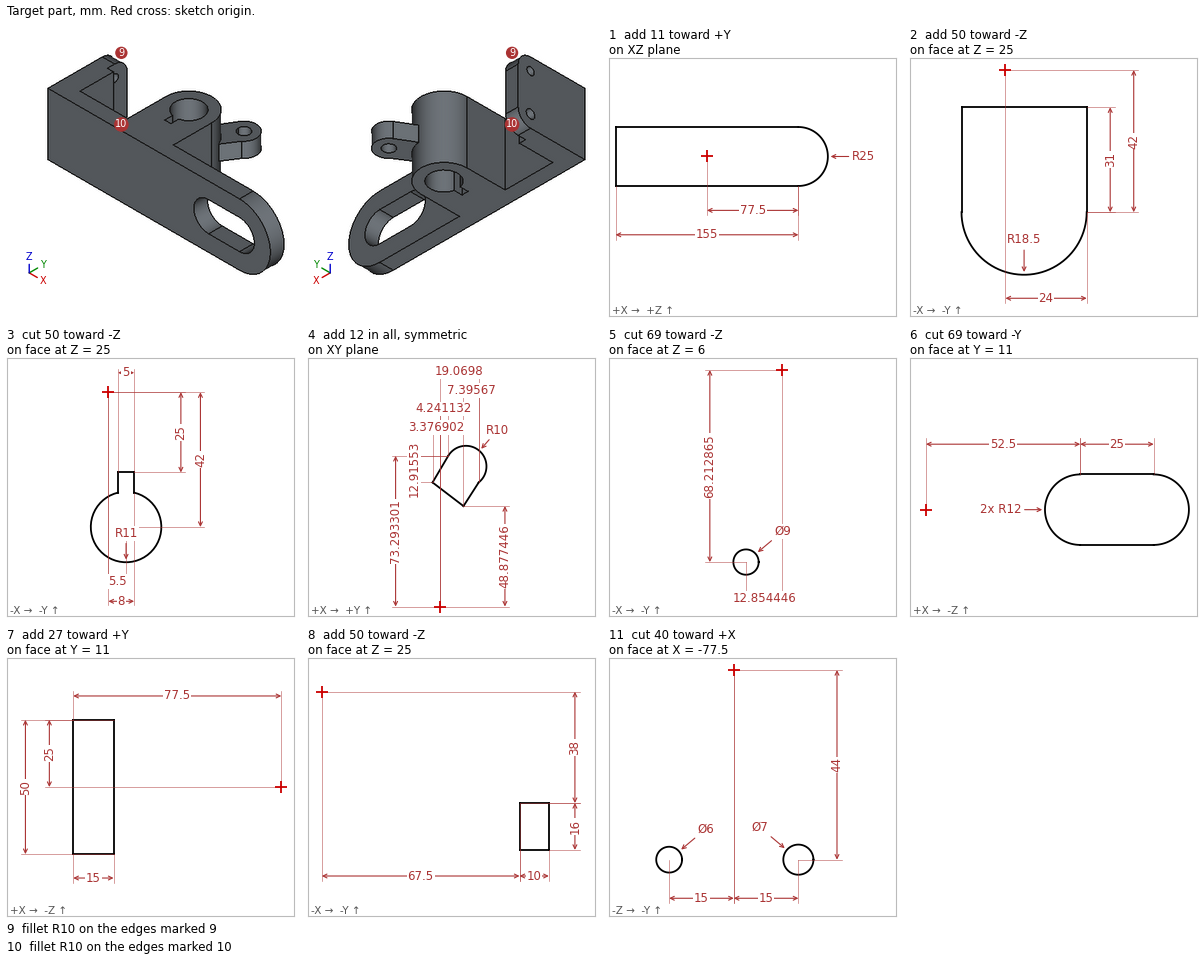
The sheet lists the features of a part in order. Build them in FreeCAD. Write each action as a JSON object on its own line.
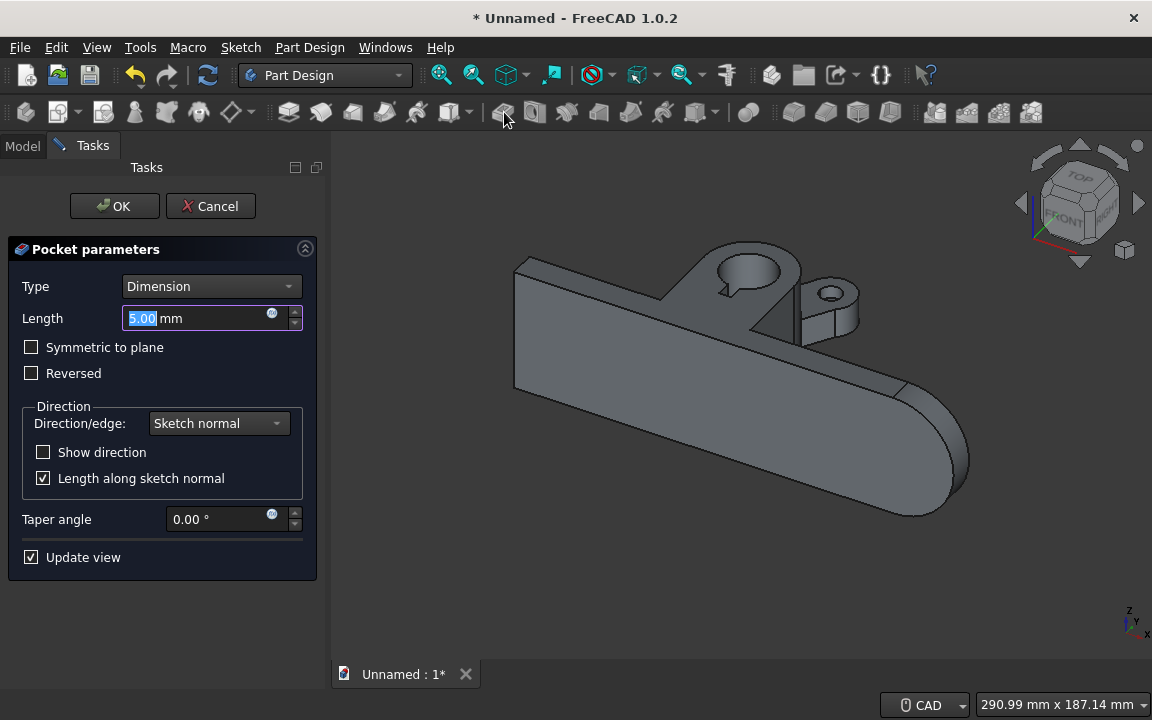
{"action": "type", "text": "69"}
{"action": "key", "text": "Tab"}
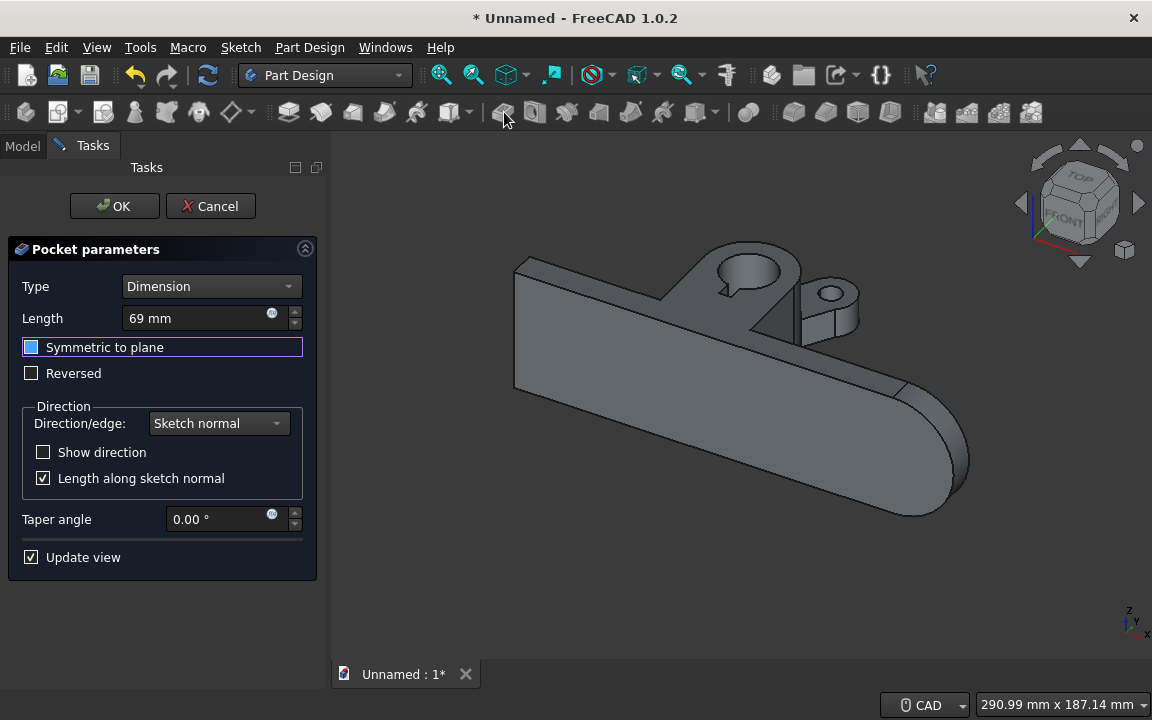
{"action": "left_click", "coordinate": [115, 206]}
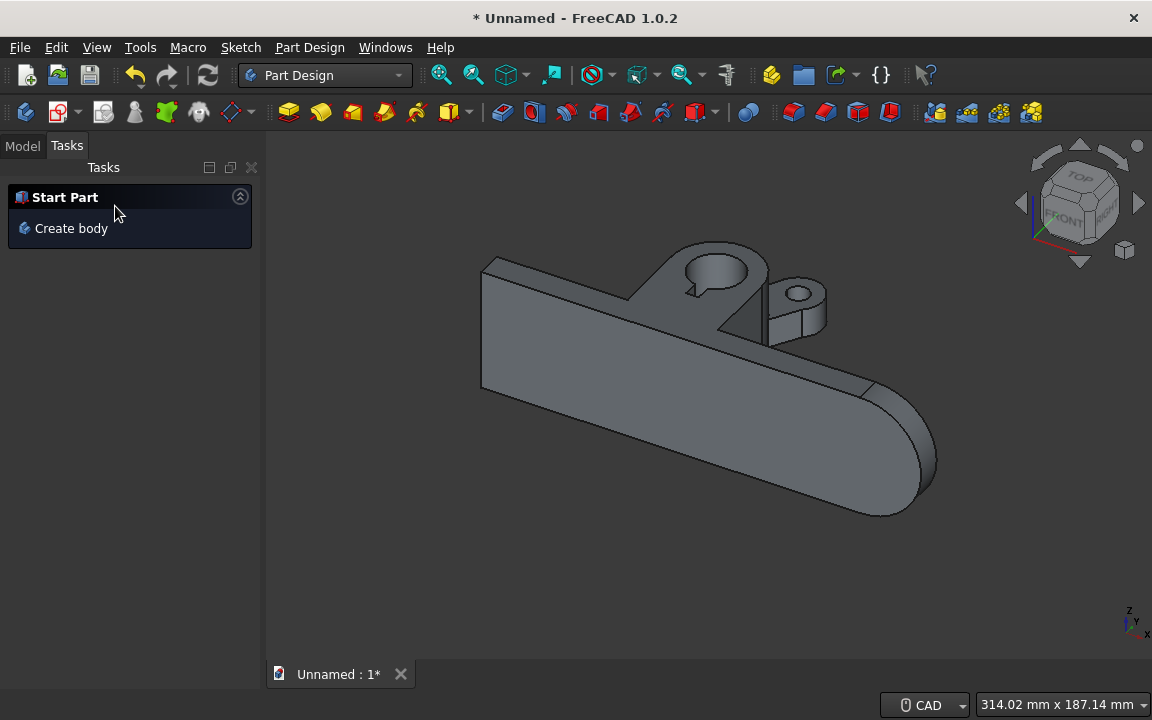
{"action": "key", "text": "4"}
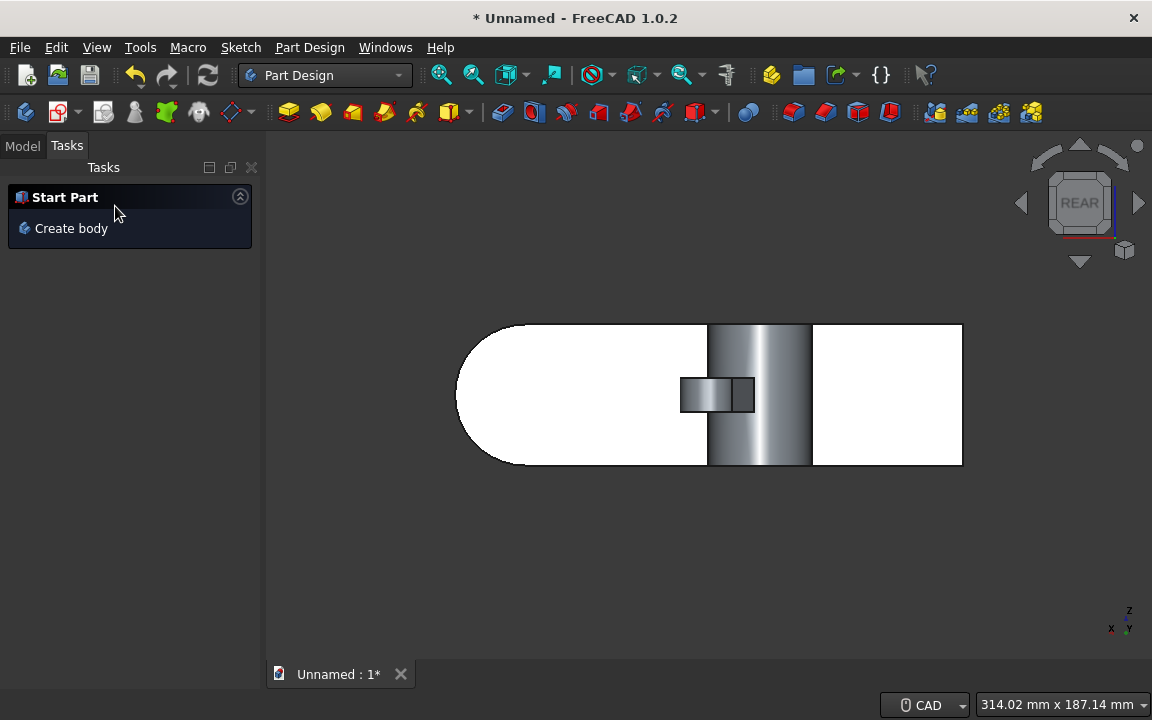
{"action": "left_click", "coordinate": [545, 394]}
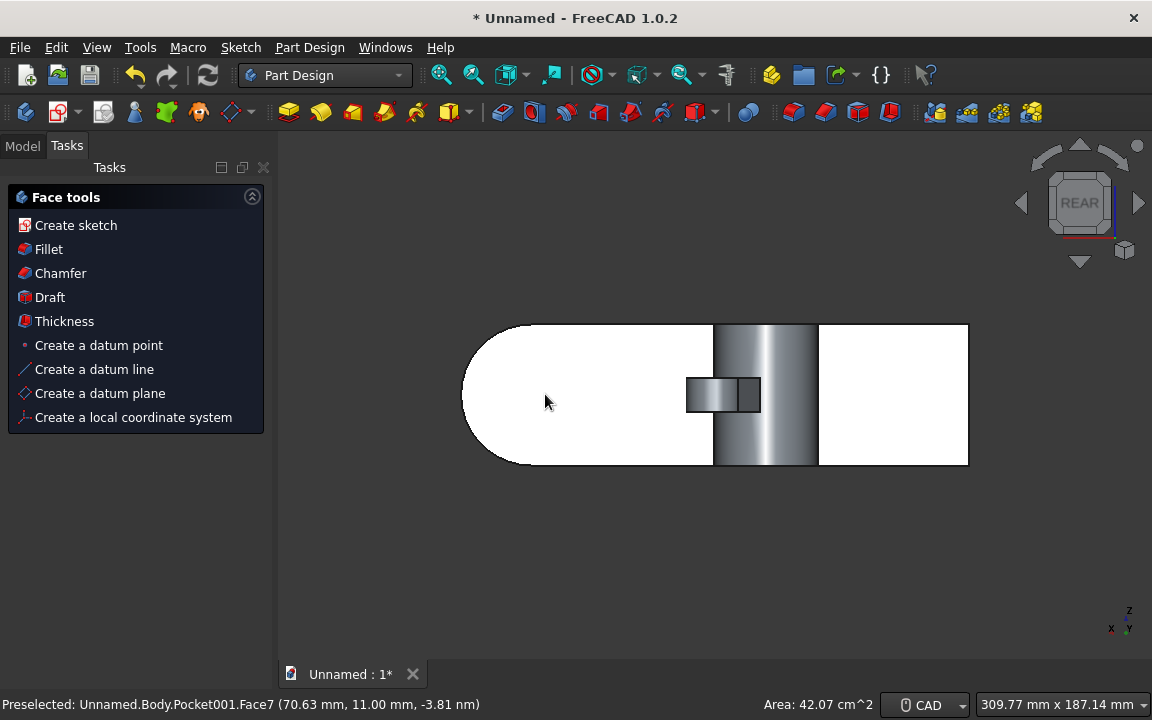
{"action": "left_click", "coordinate": [58, 112]}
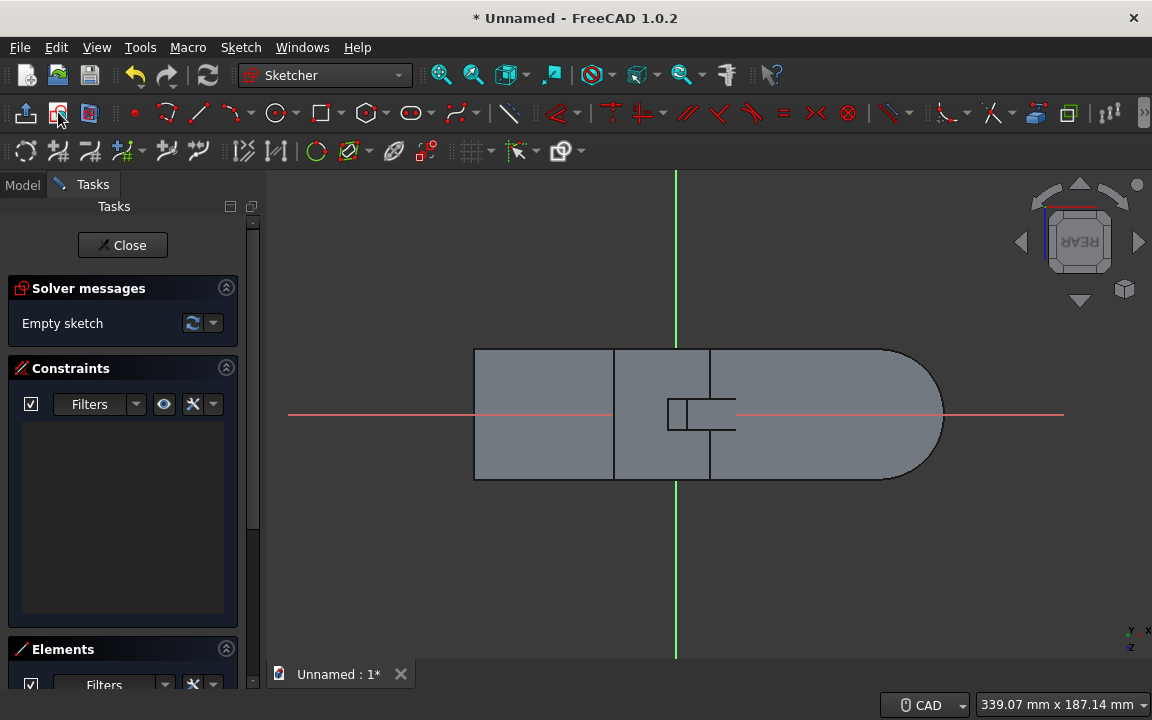
{"action": "left_click", "coordinate": [90, 114]}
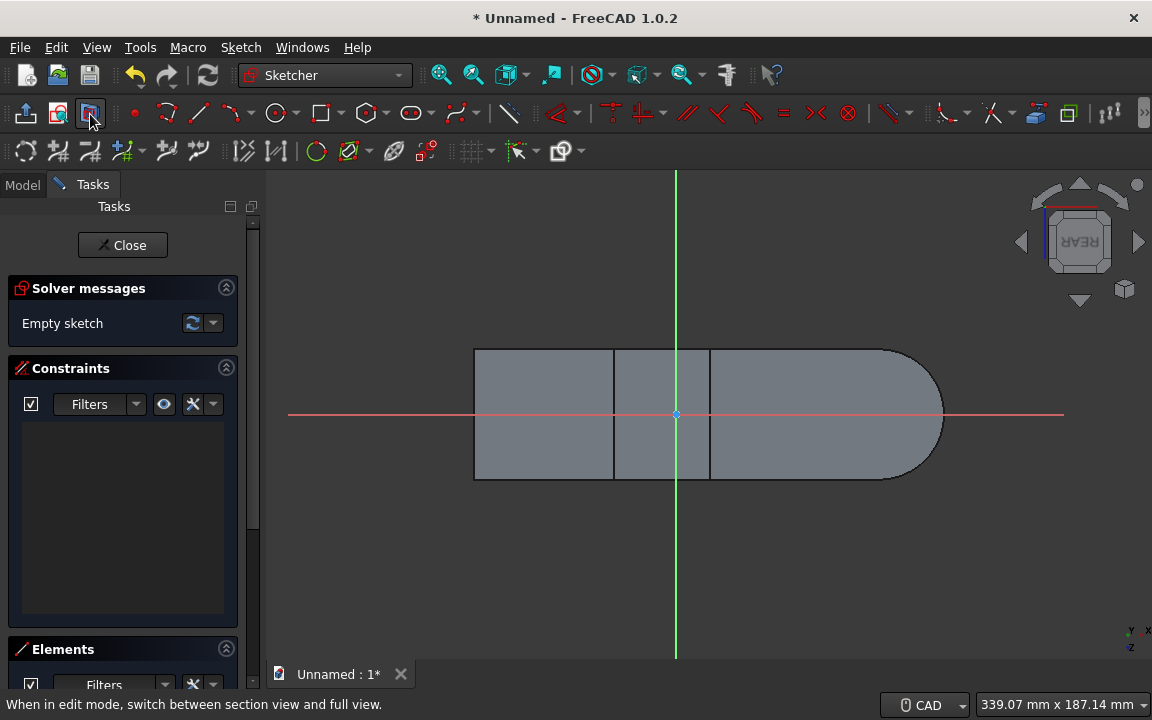
{"action": "scroll", "coordinate": [918, 415], "scroll_direction": "up", "scroll_amount": 4}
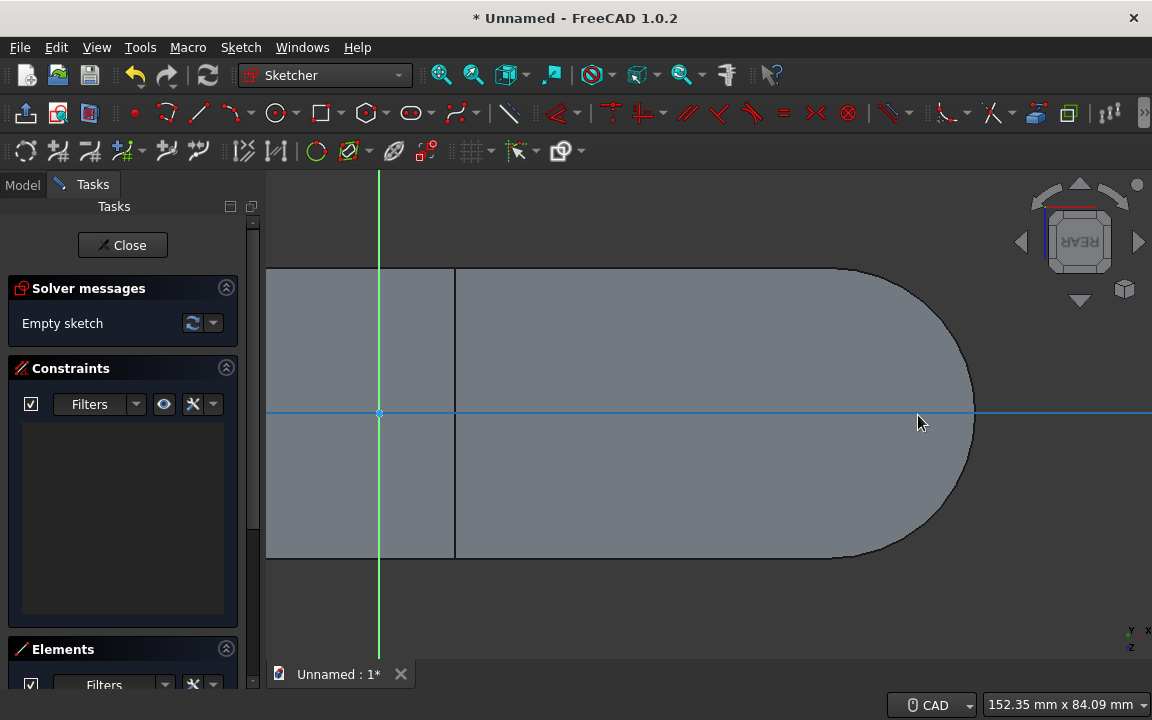
{"action": "left_click", "coordinate": [412, 114]}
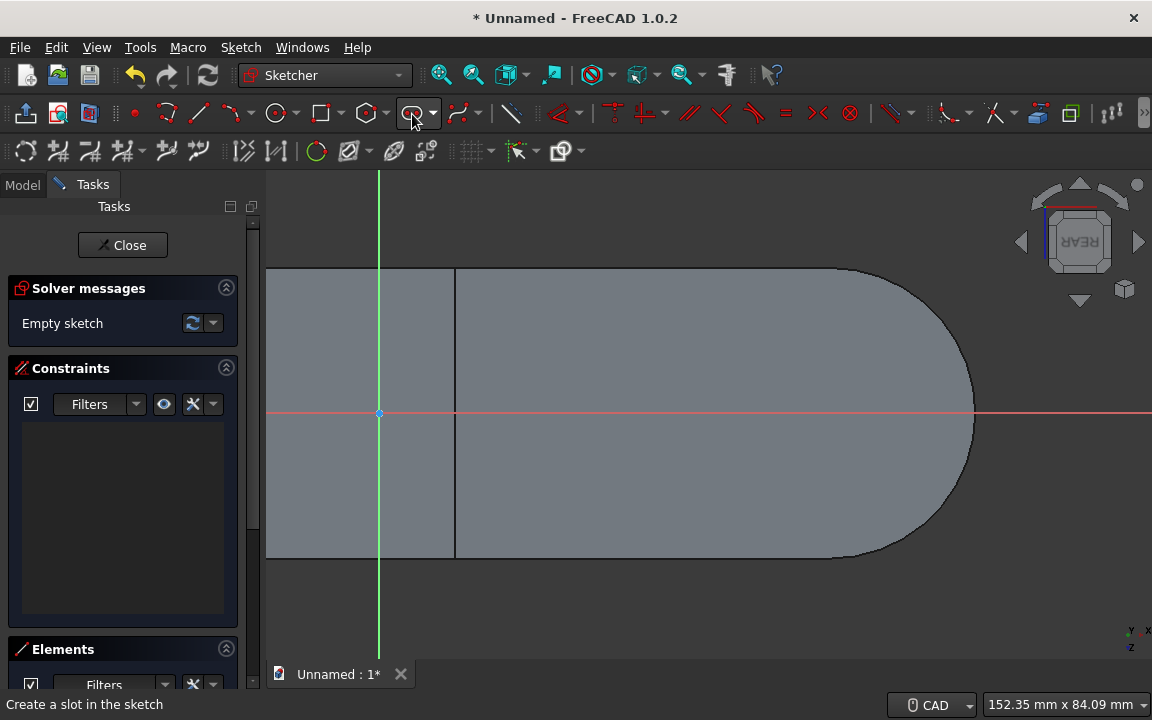
{"action": "left_click", "coordinate": [685, 413]}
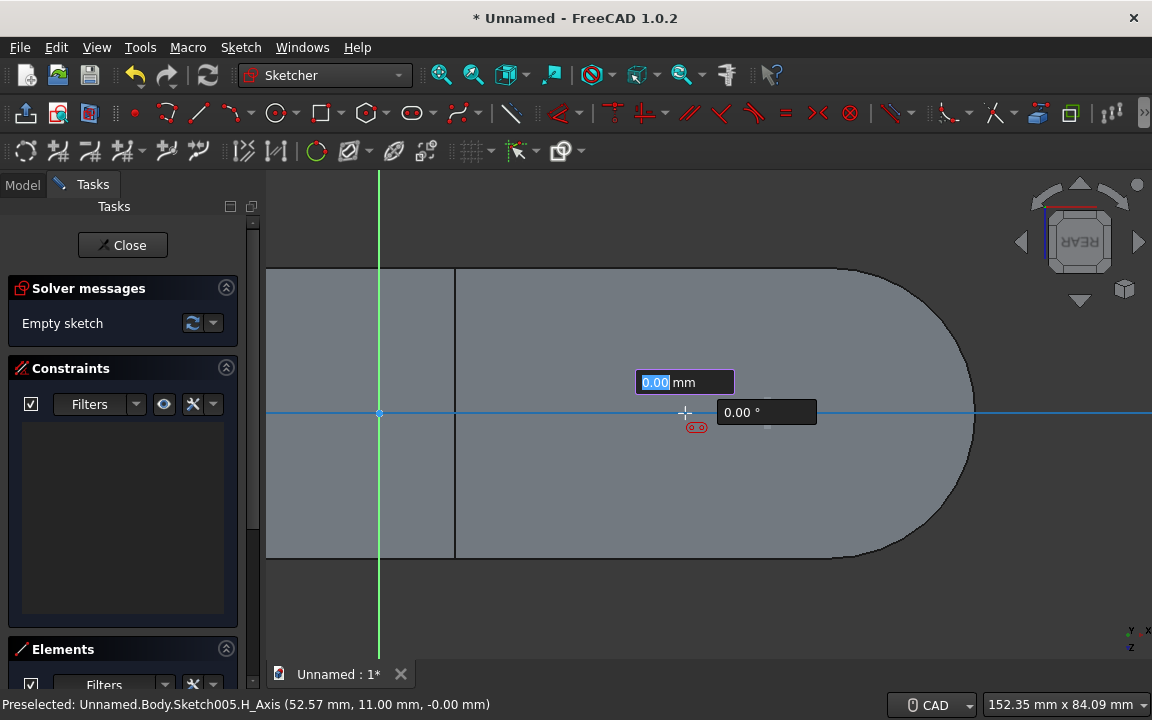
{"action": "left_click", "coordinate": [830, 404]}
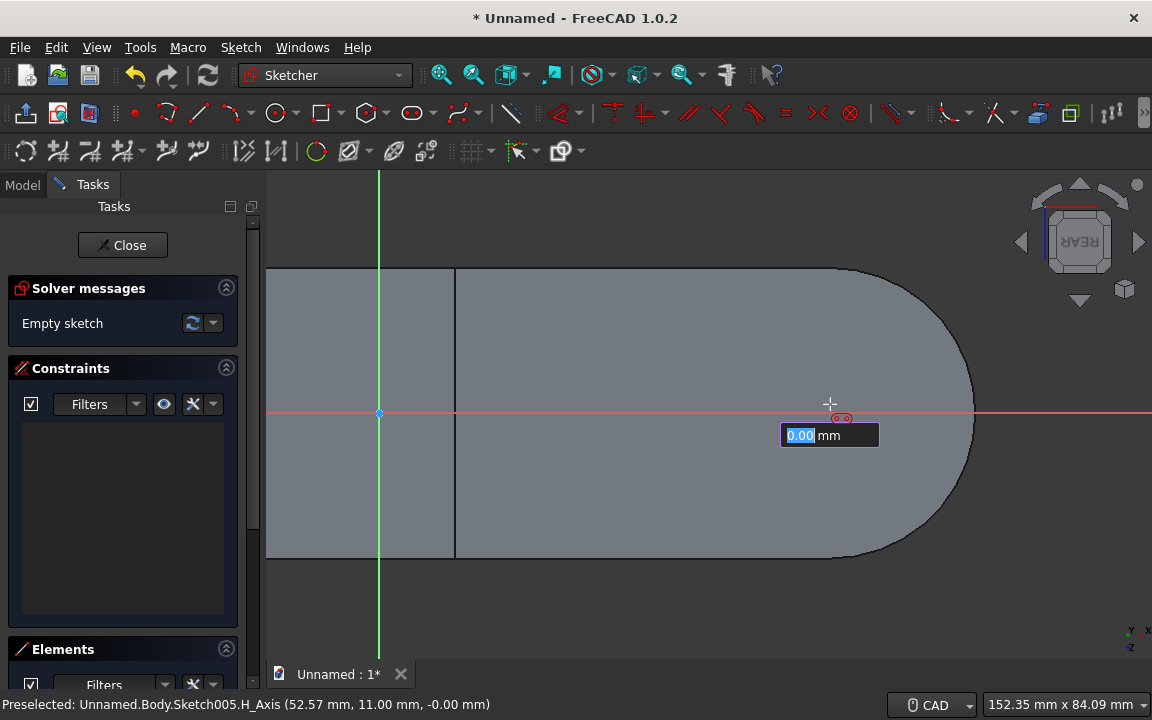
{"action": "left_click", "coordinate": [757, 343]}
{"action": "key", "text": "Escape"}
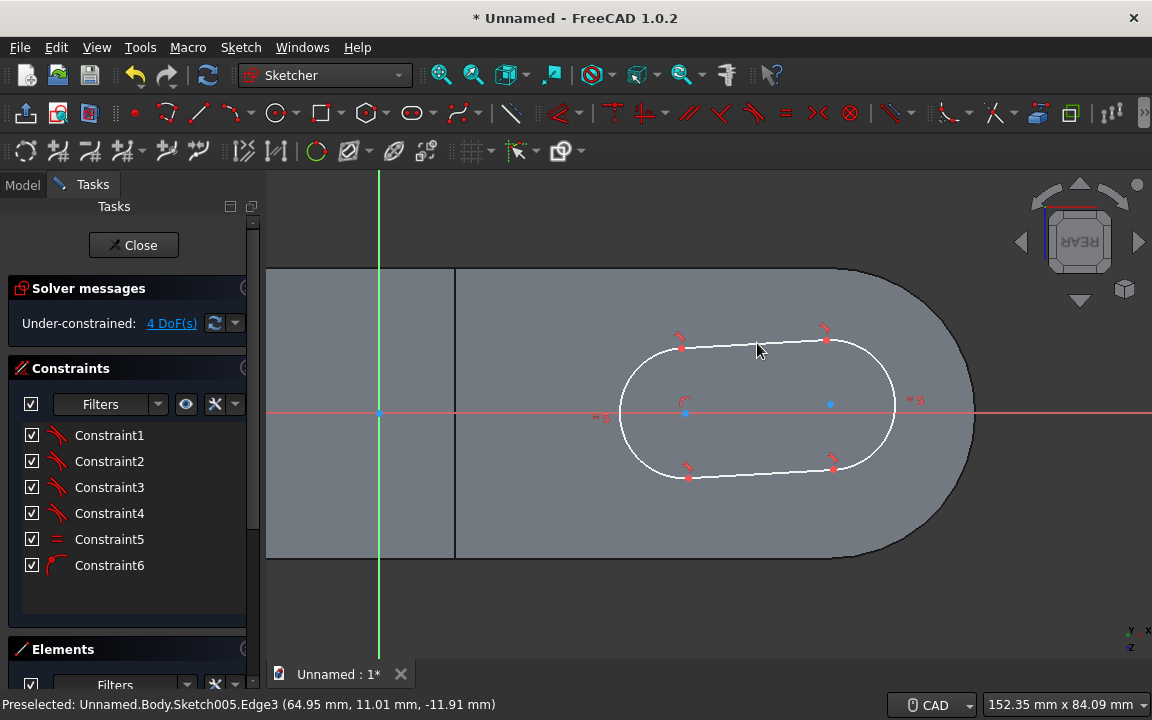
{"action": "left_click", "coordinate": [725, 346]}